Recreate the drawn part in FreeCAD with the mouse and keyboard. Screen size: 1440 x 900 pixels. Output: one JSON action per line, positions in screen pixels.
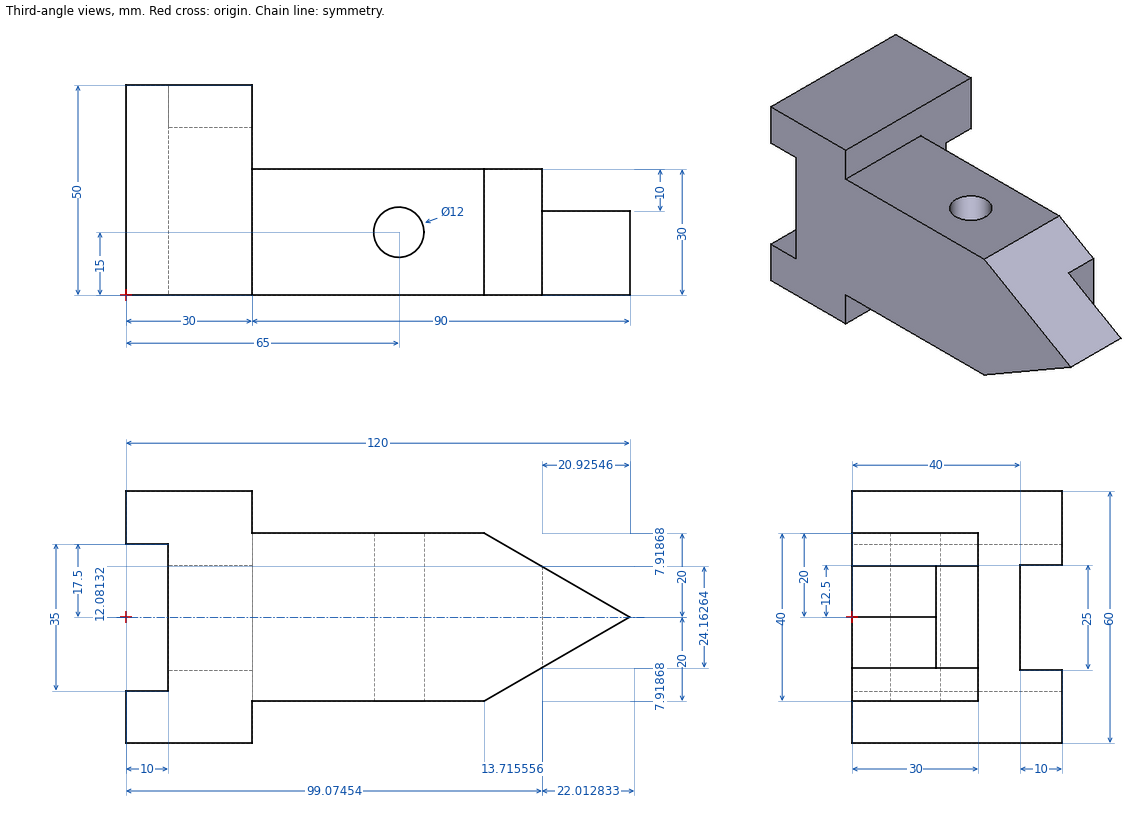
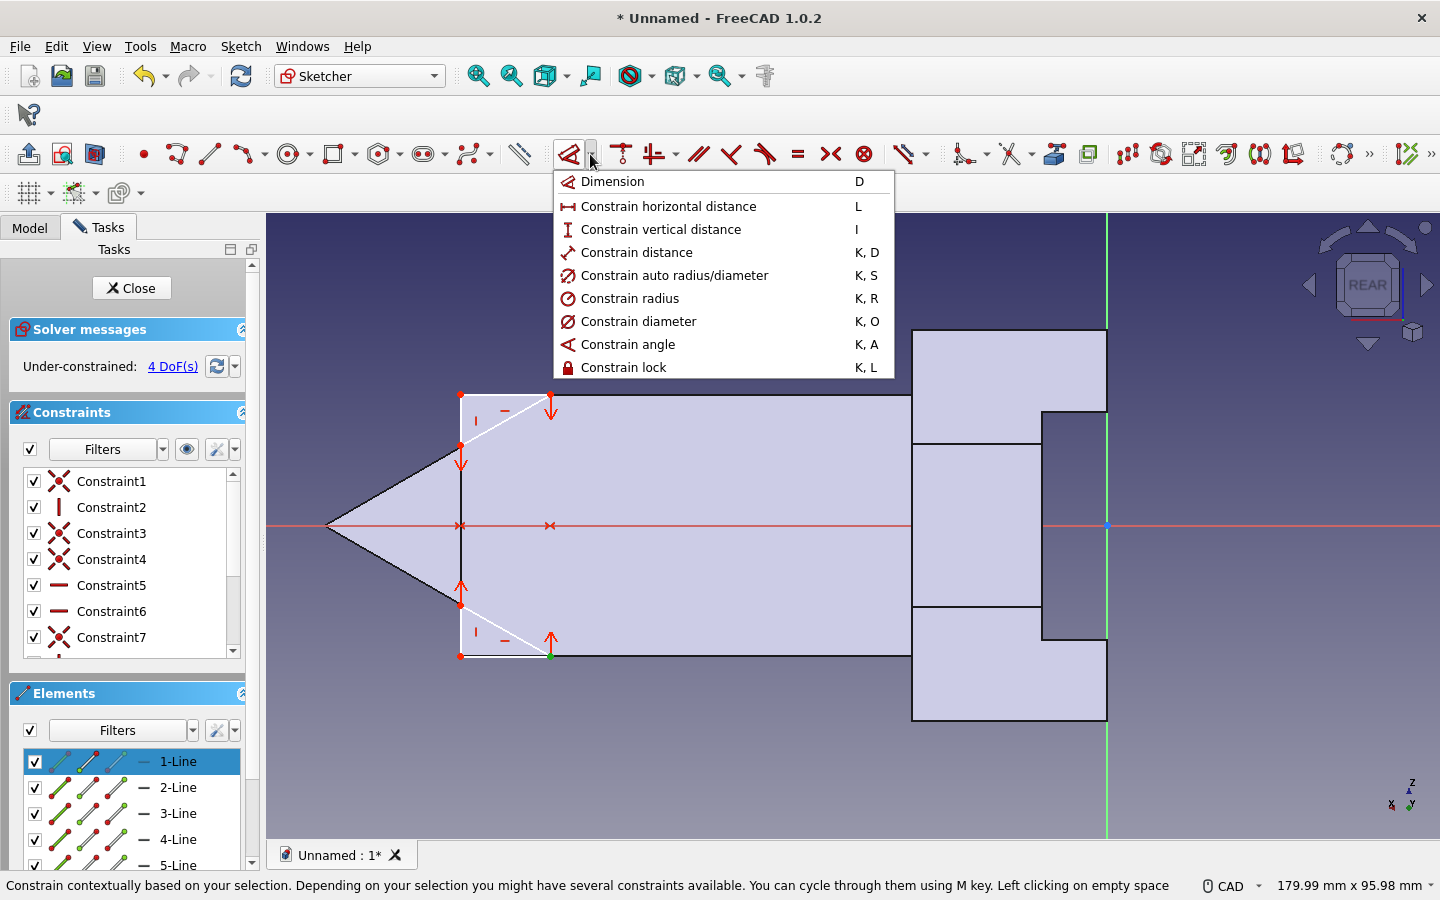
{"action": "left_click", "coordinate": [724, 230]}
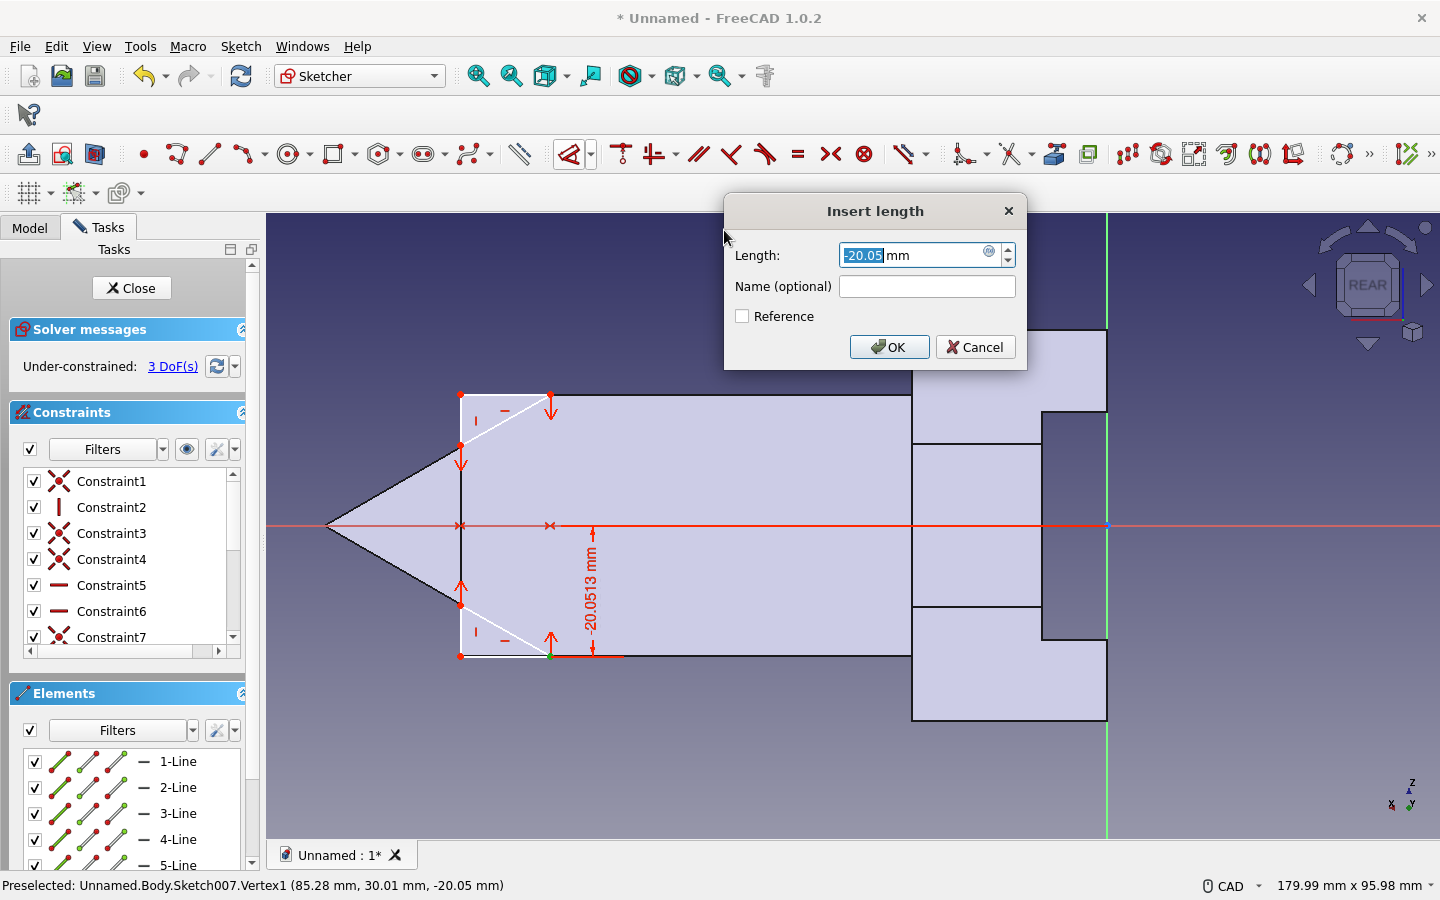
{"action": "type", "text": "-20"}
{"action": "key", "text": "Return"}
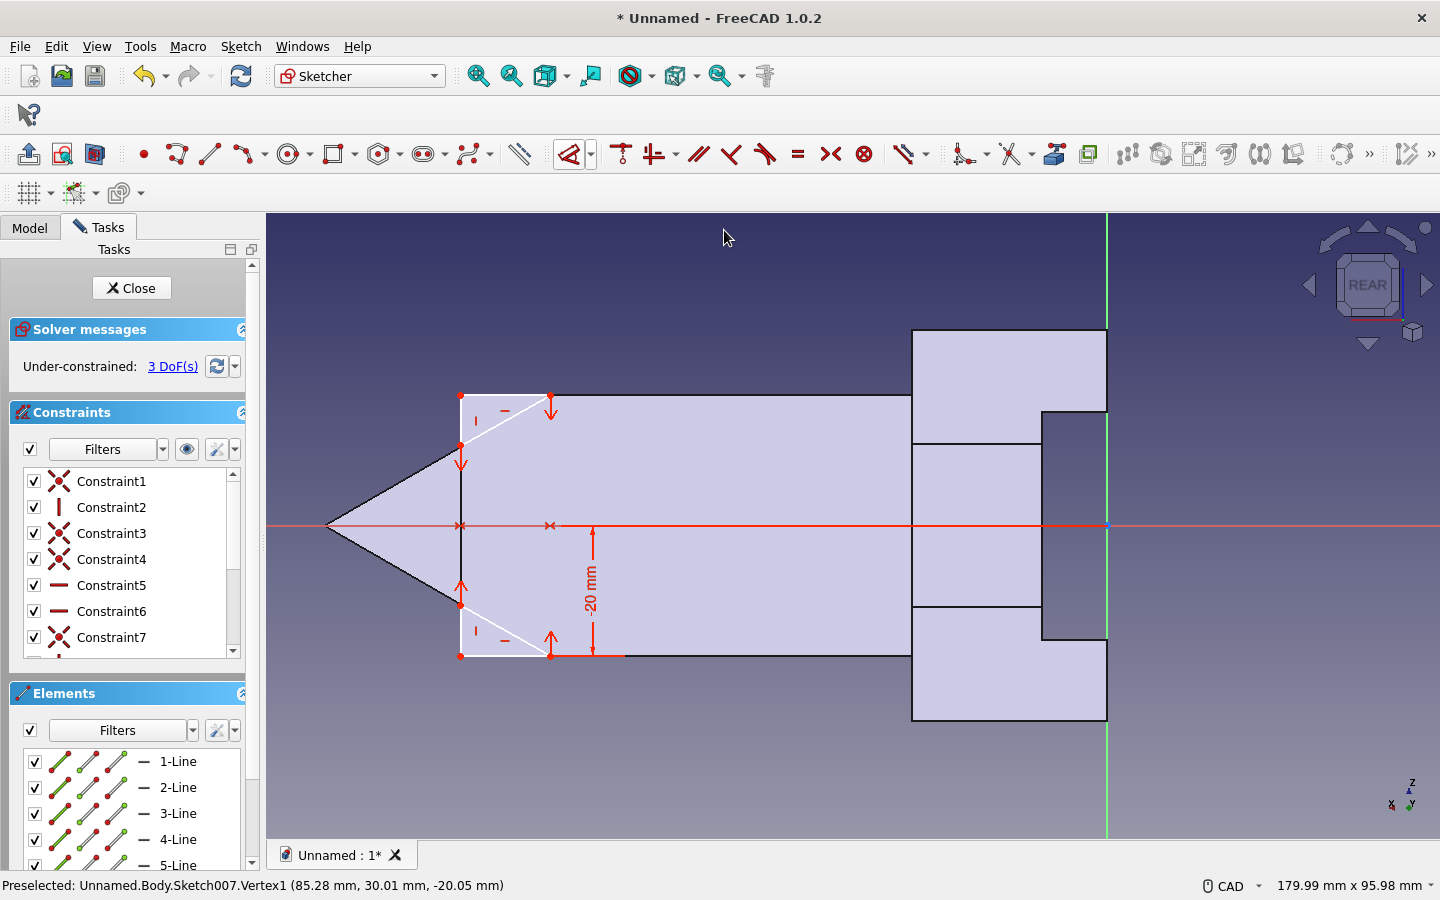
{"action": "left_click", "coordinate": [461, 621]}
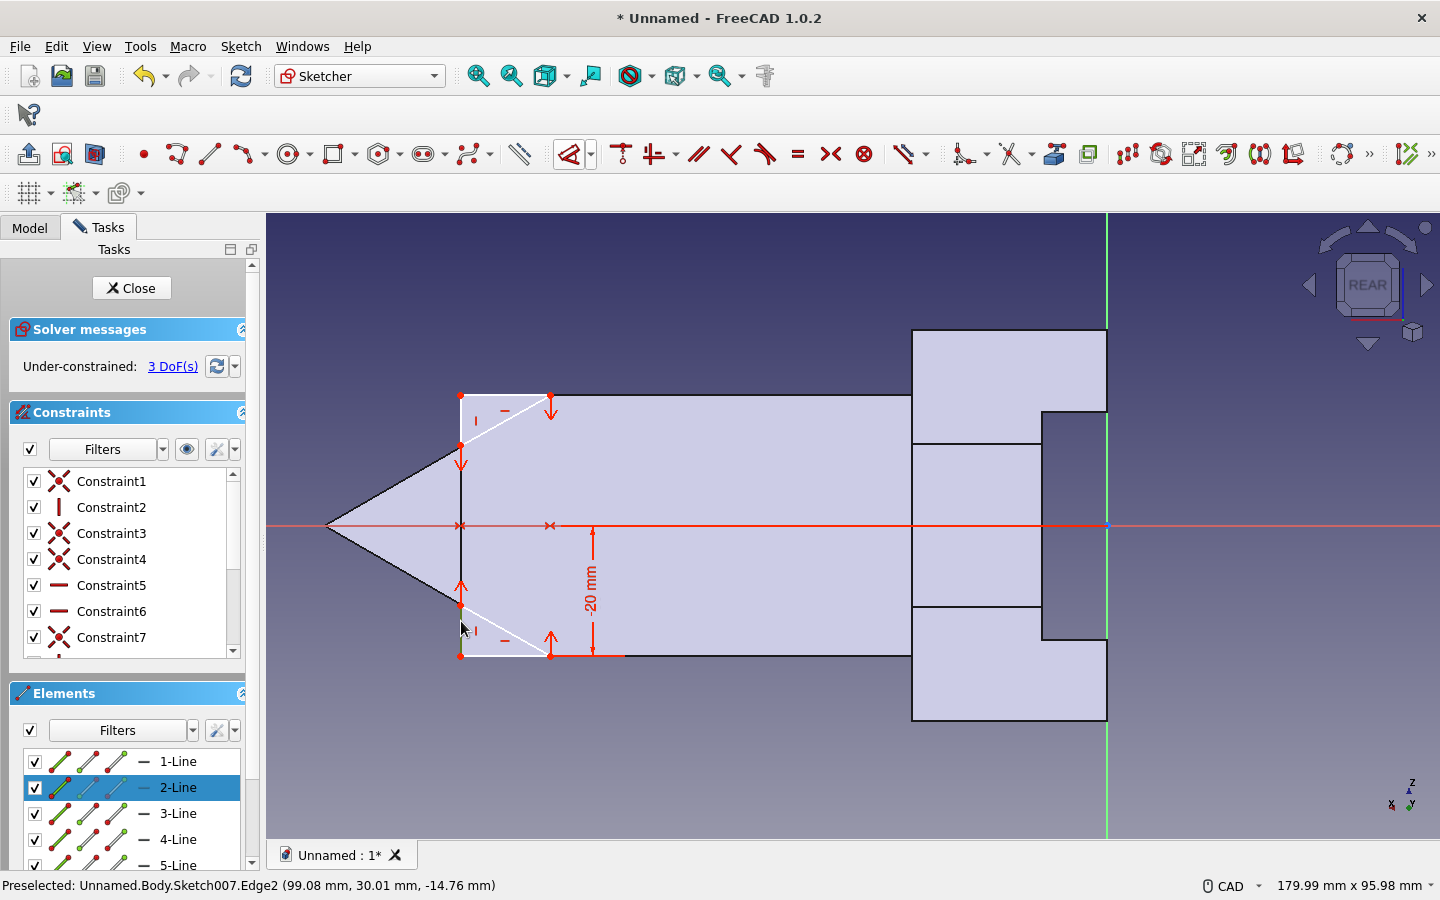
{"action": "key", "text": "i"}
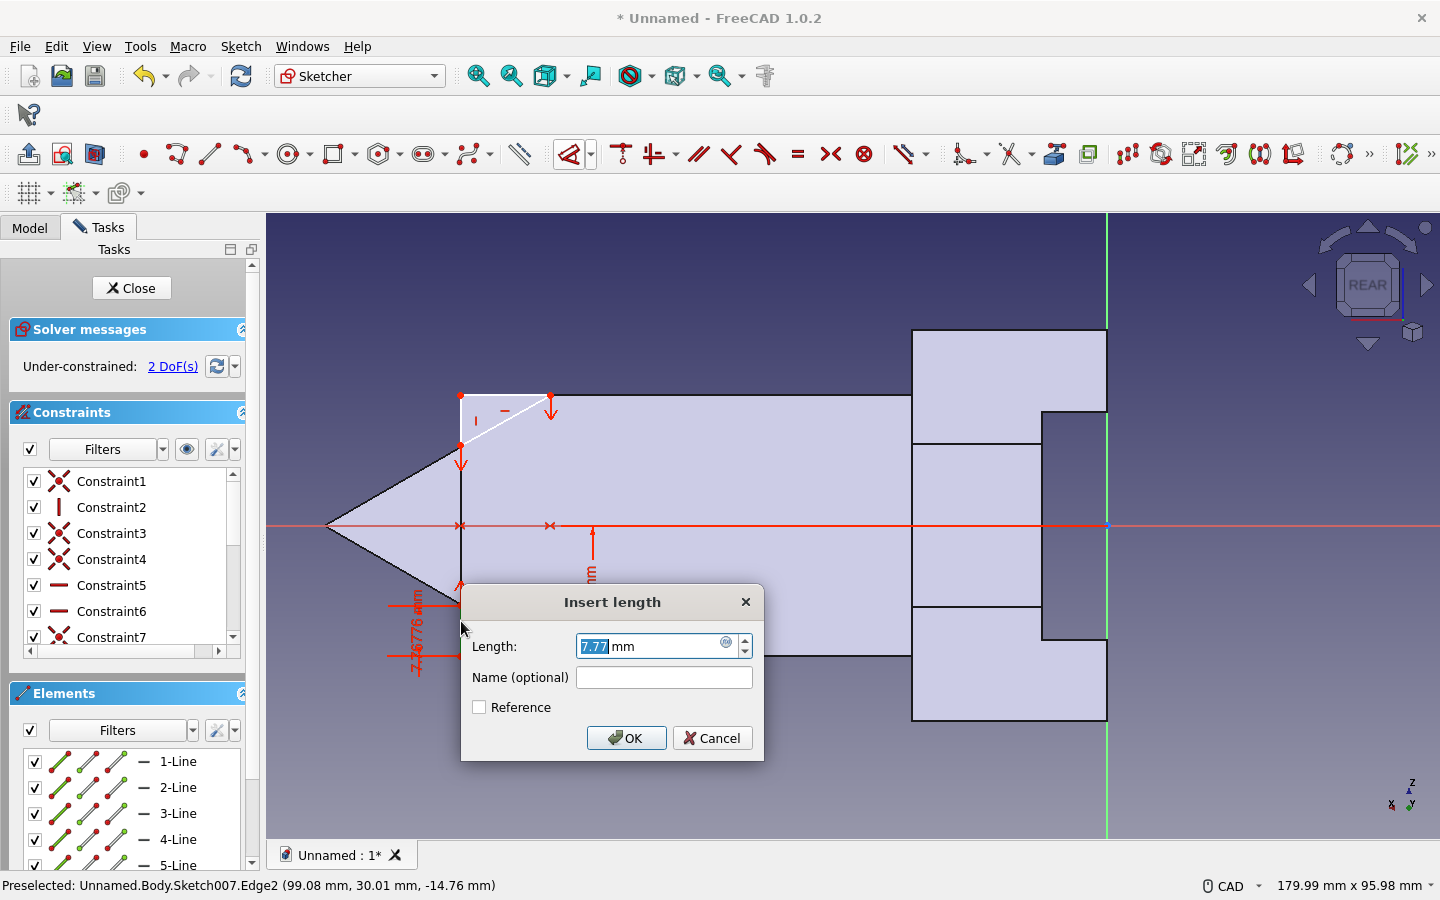
{"action": "type", "text": "7.91868"}
{"action": "key", "text": "Return"}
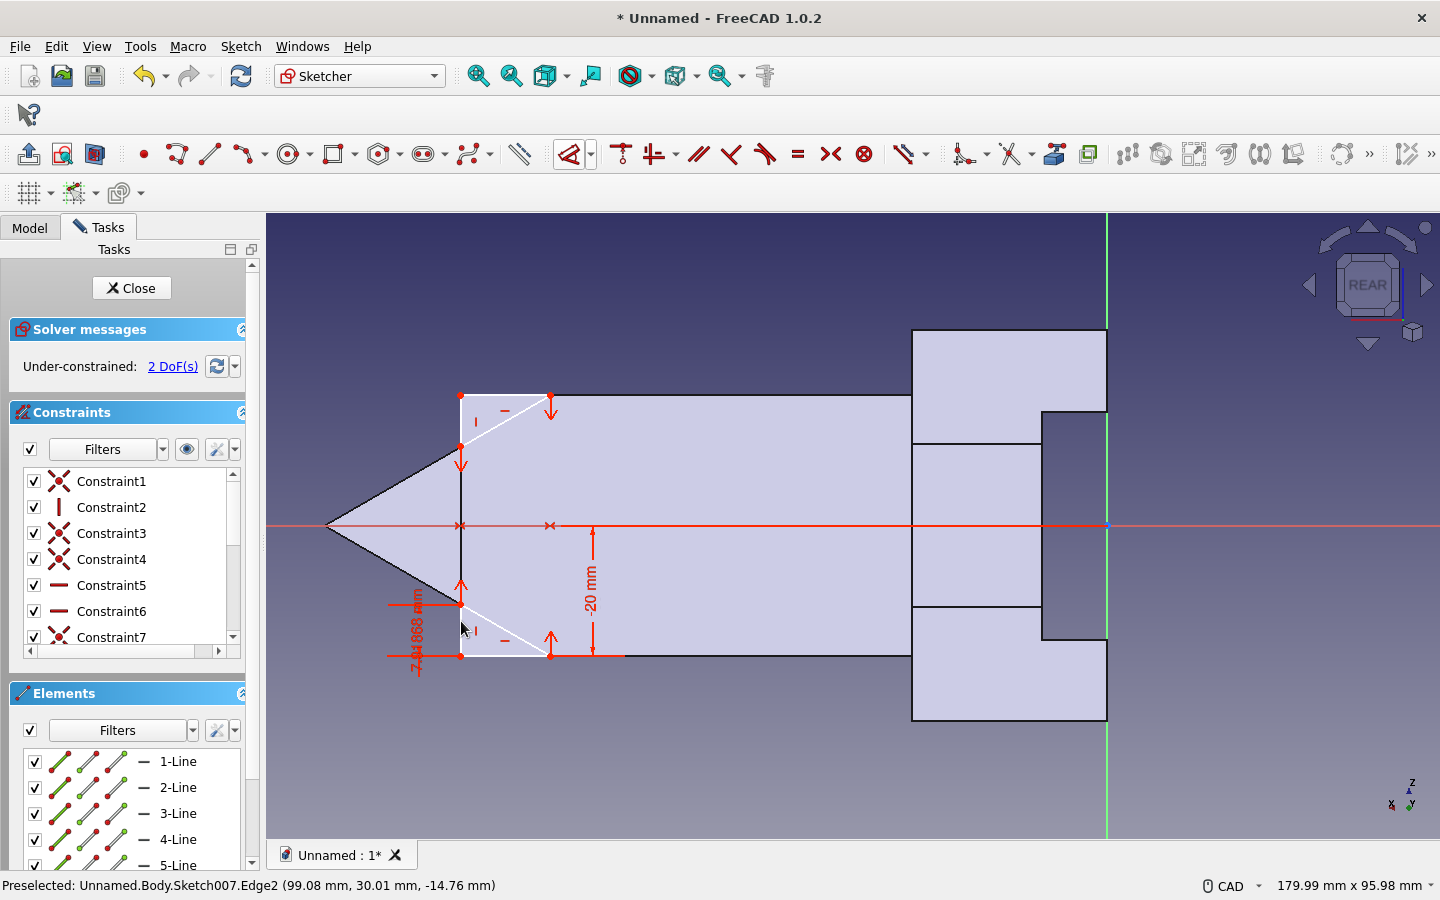
{"action": "left_click", "coordinate": [488, 656]}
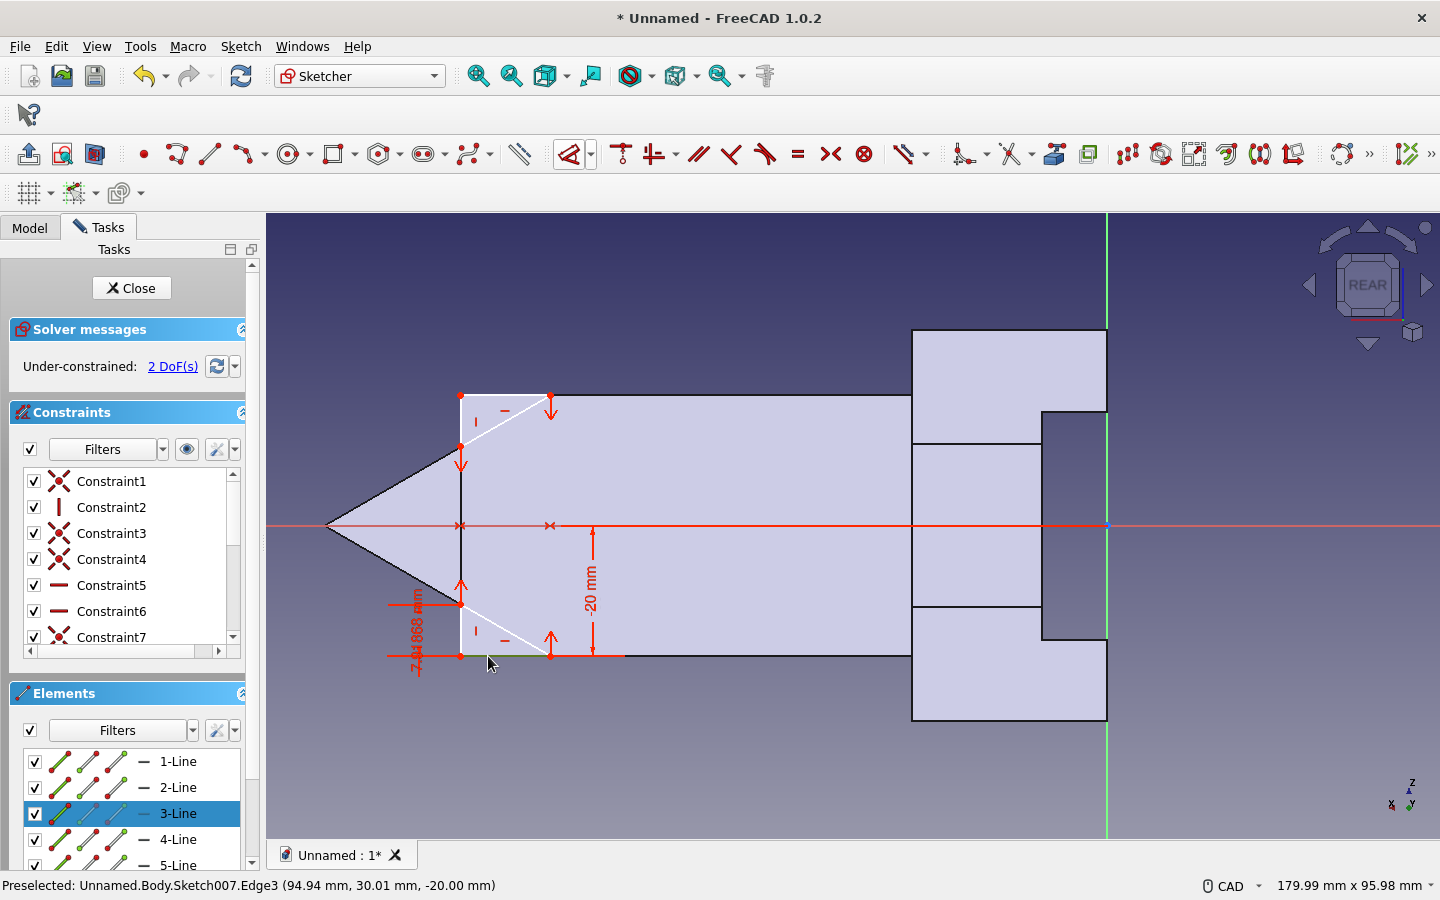
{"action": "key", "text": "l"}